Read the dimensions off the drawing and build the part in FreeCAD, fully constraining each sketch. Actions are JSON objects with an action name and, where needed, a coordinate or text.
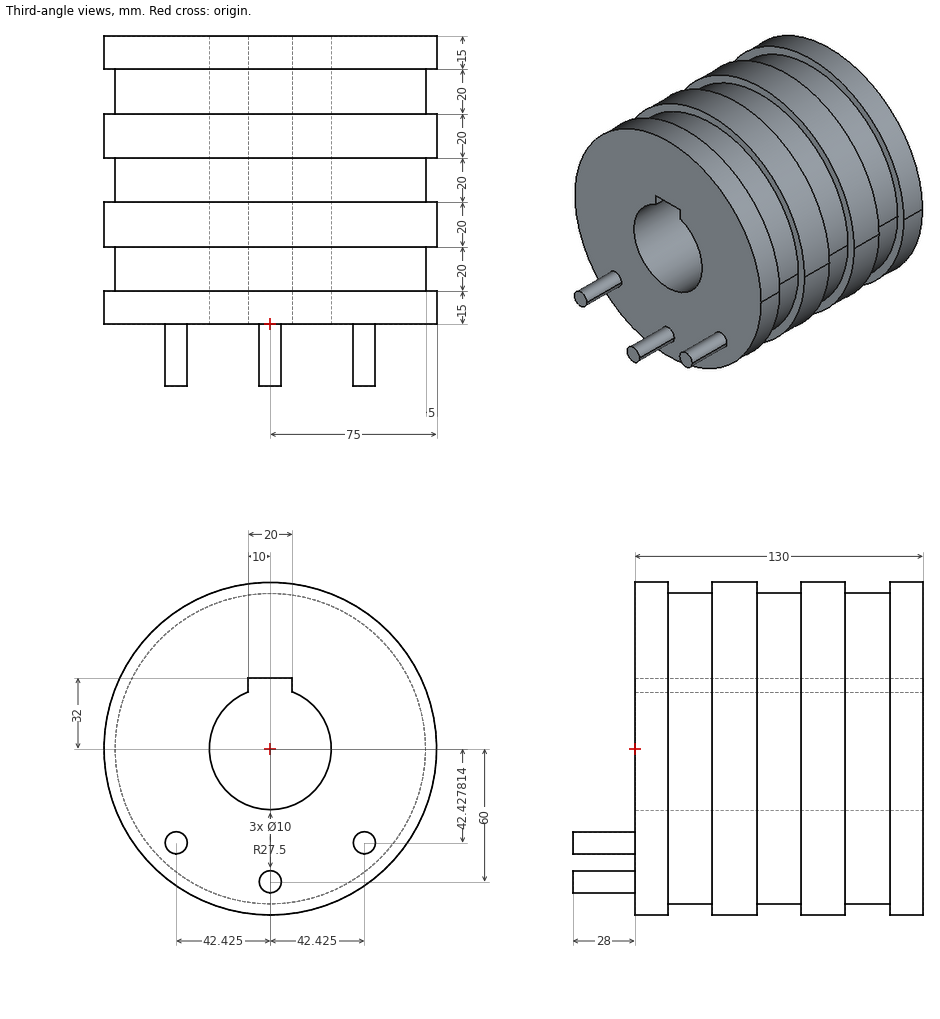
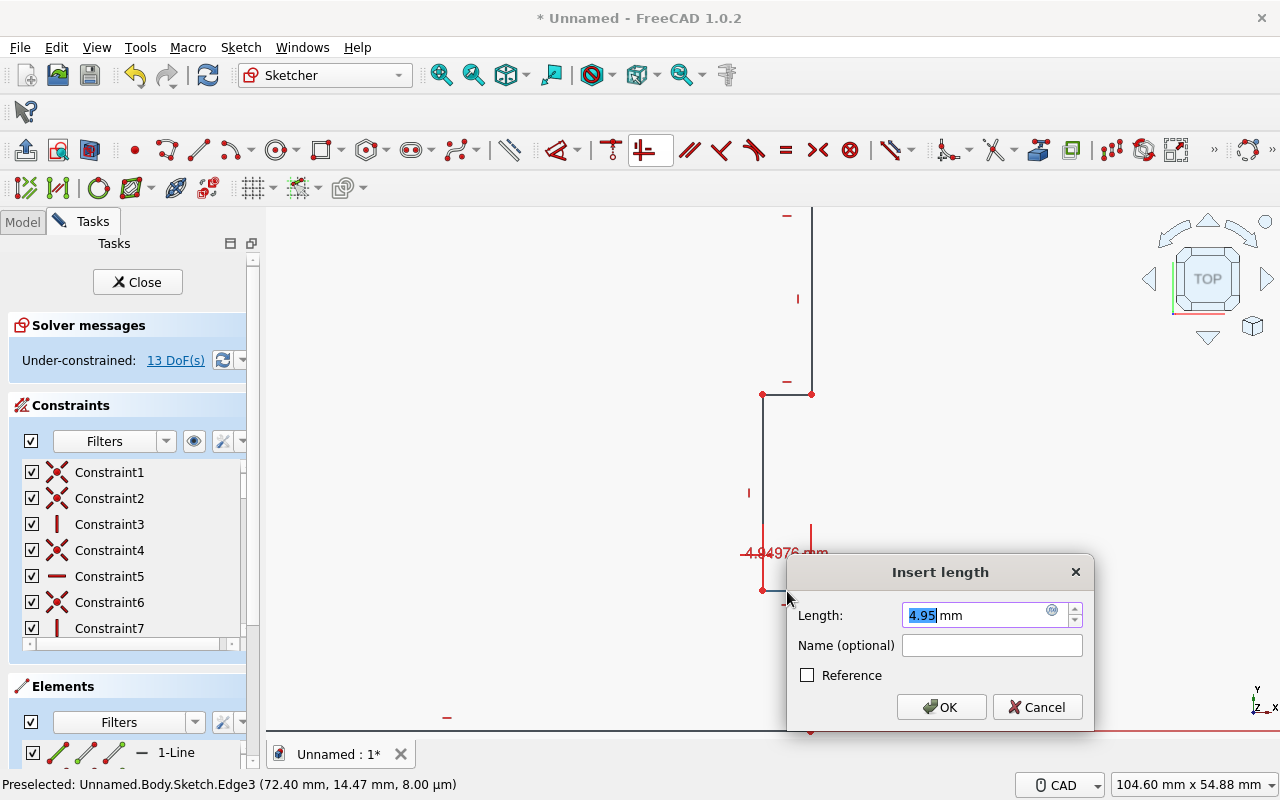
{"action": "type", "text": "5"}
{"action": "key", "text": "Return"}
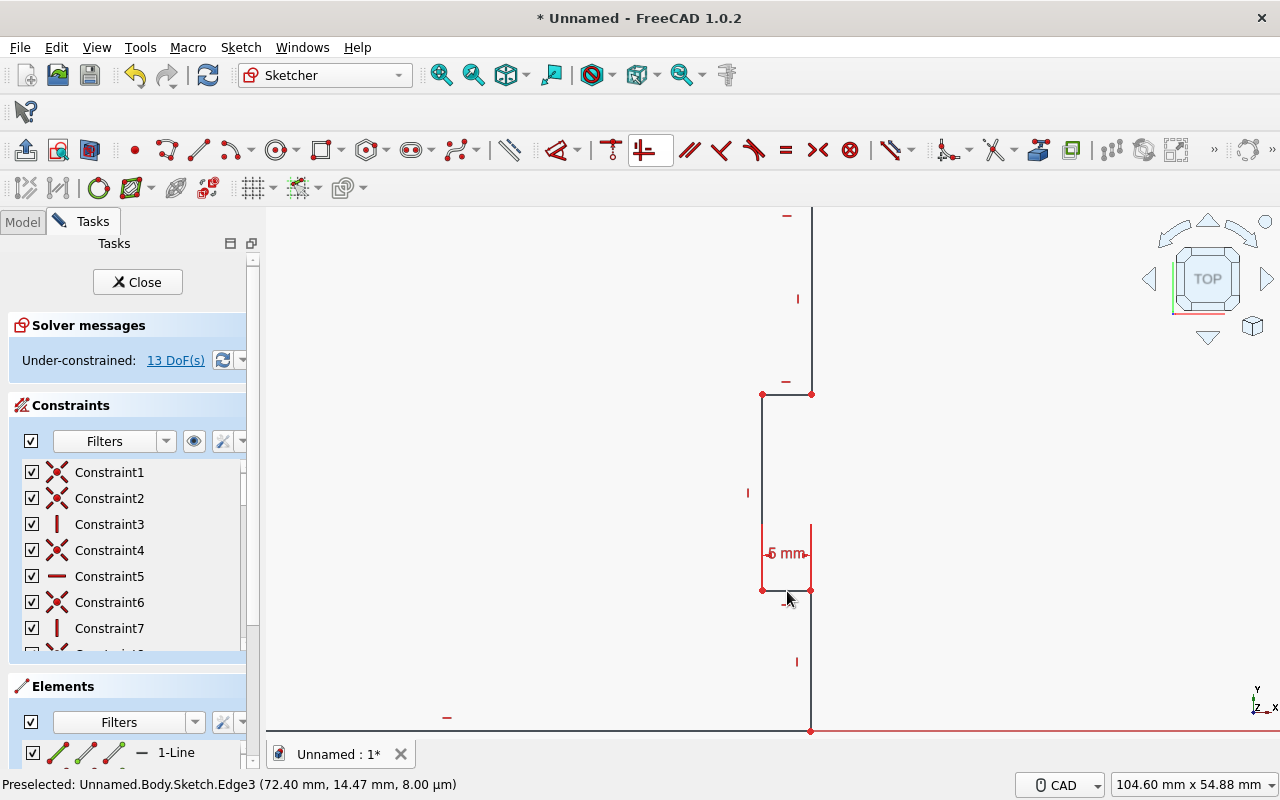
{"action": "left_click", "coordinate": [777, 395]}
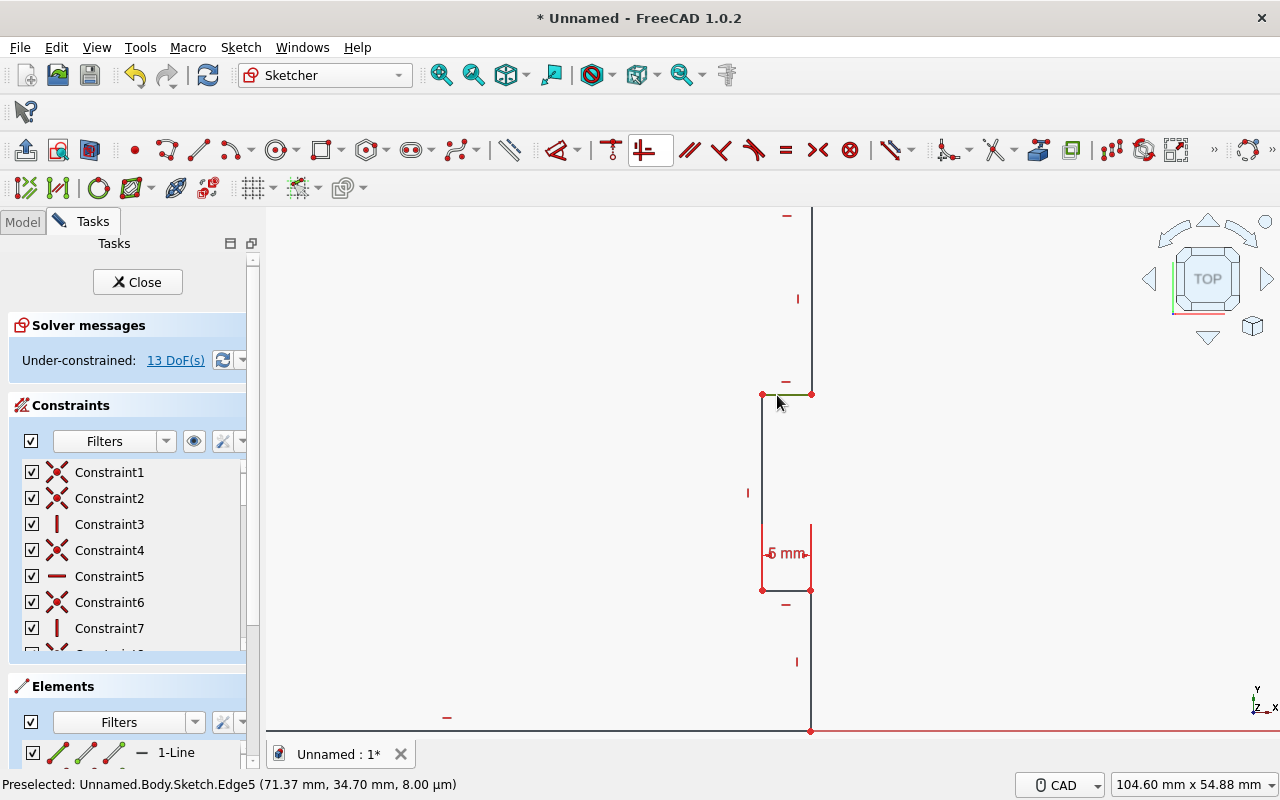
{"action": "left_click", "coordinate": [580, 150]}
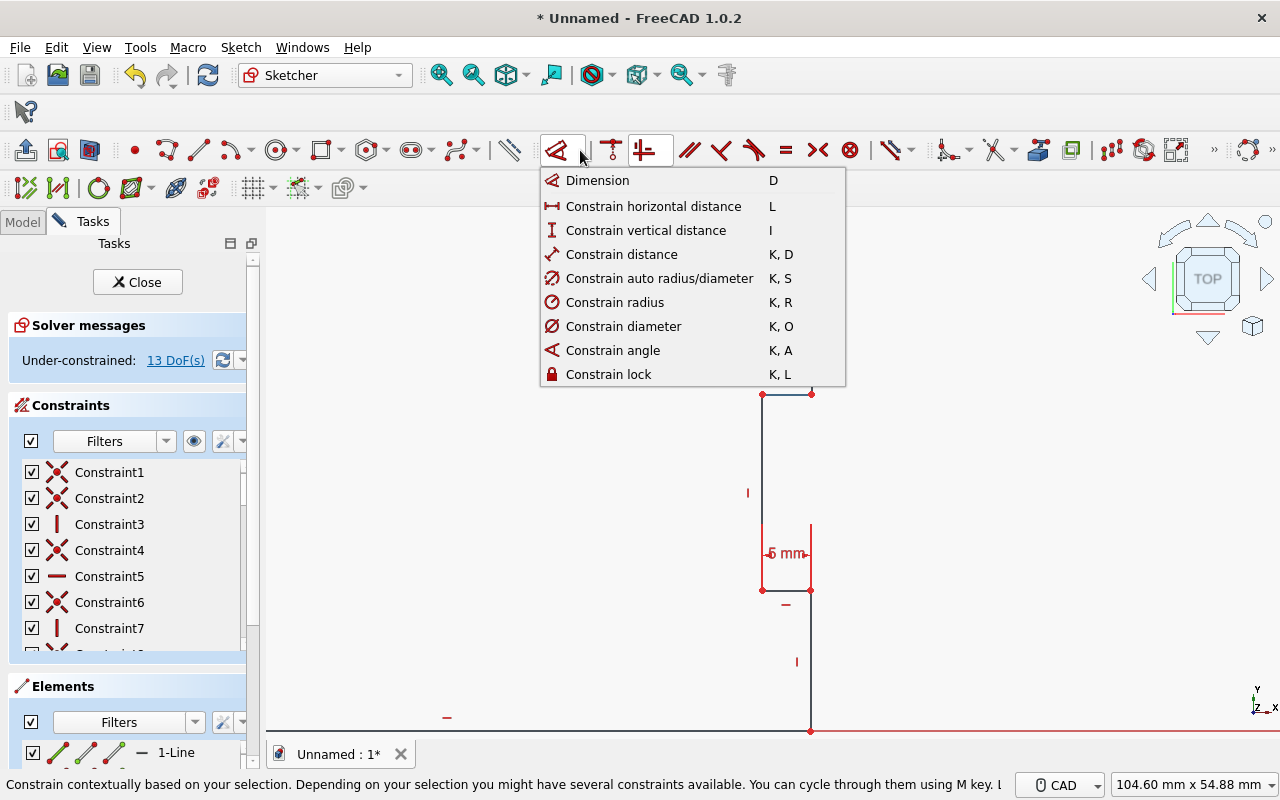
{"action": "left_click", "coordinate": [693, 206]}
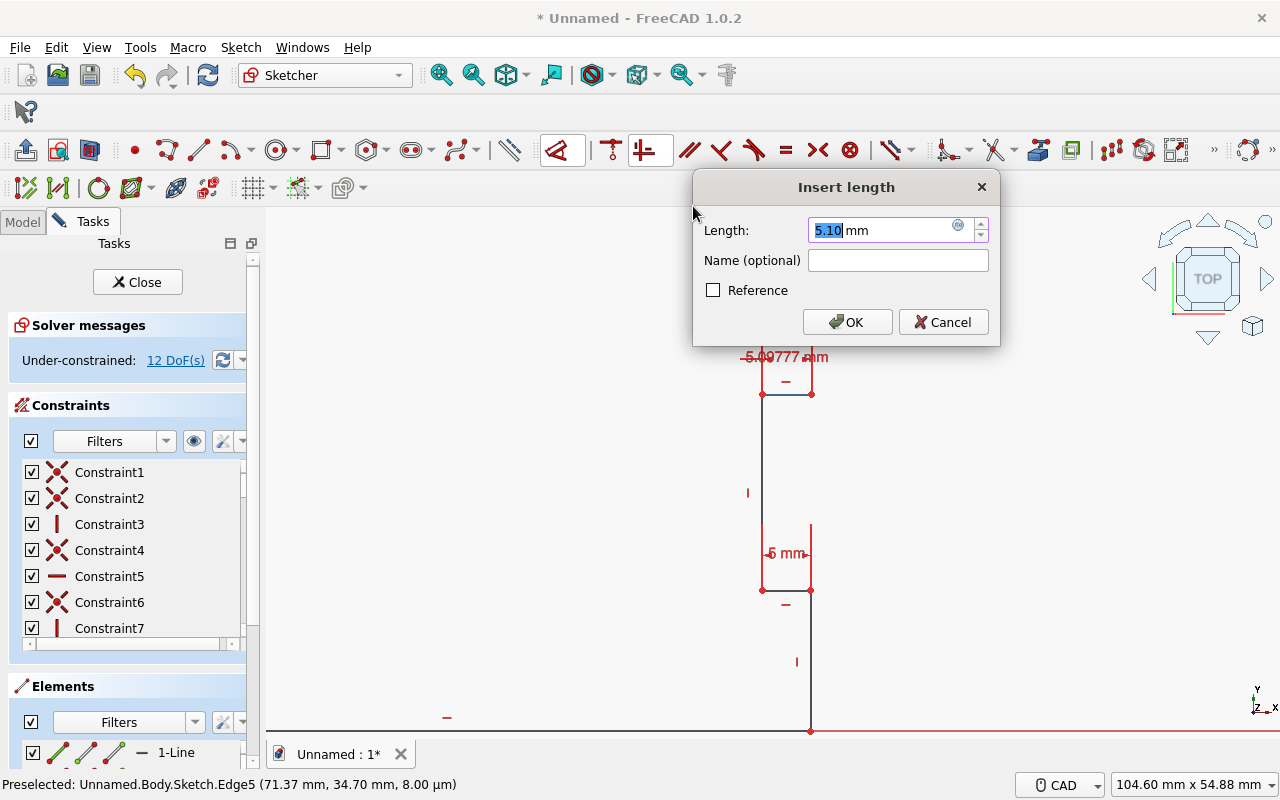
{"action": "type", "text": "5"}
{"action": "key", "text": "Return"}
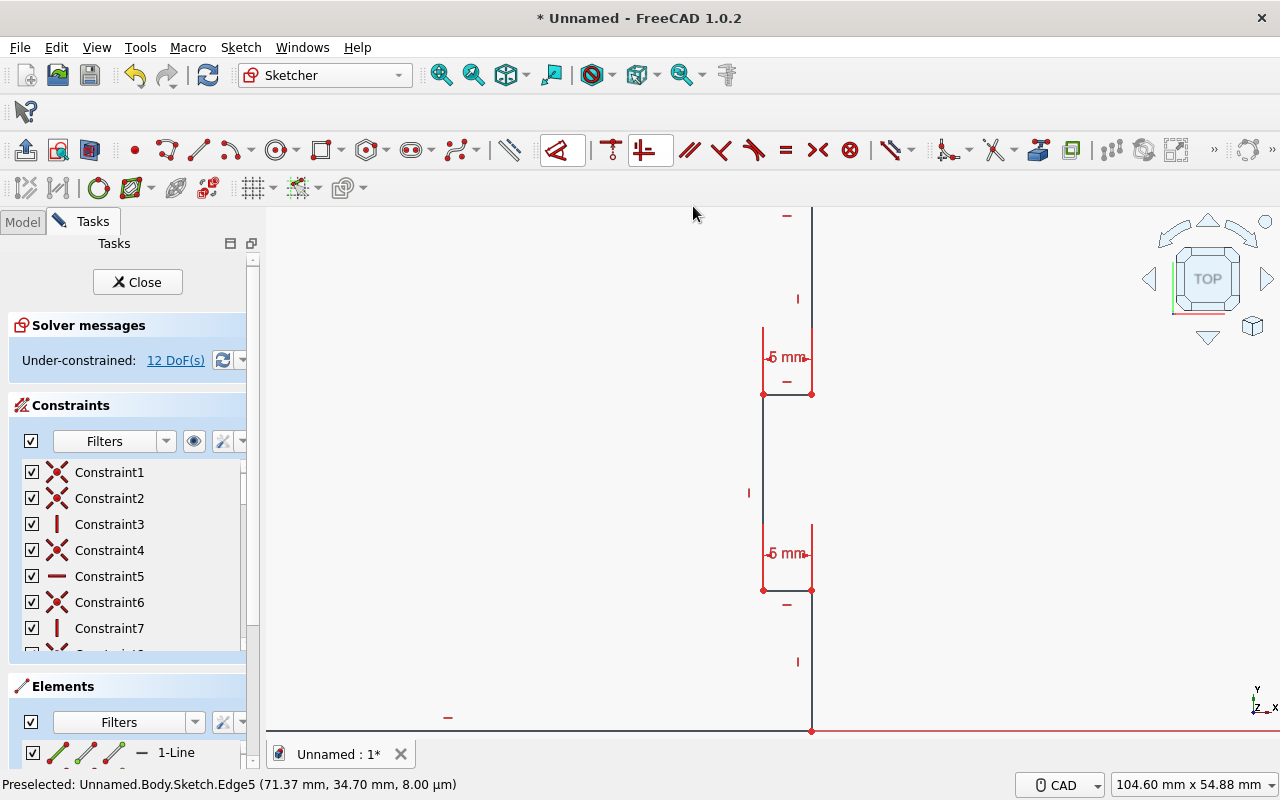
{"action": "scroll", "coordinate": [788, 595], "scroll_direction": "down", "scroll_amount": 7}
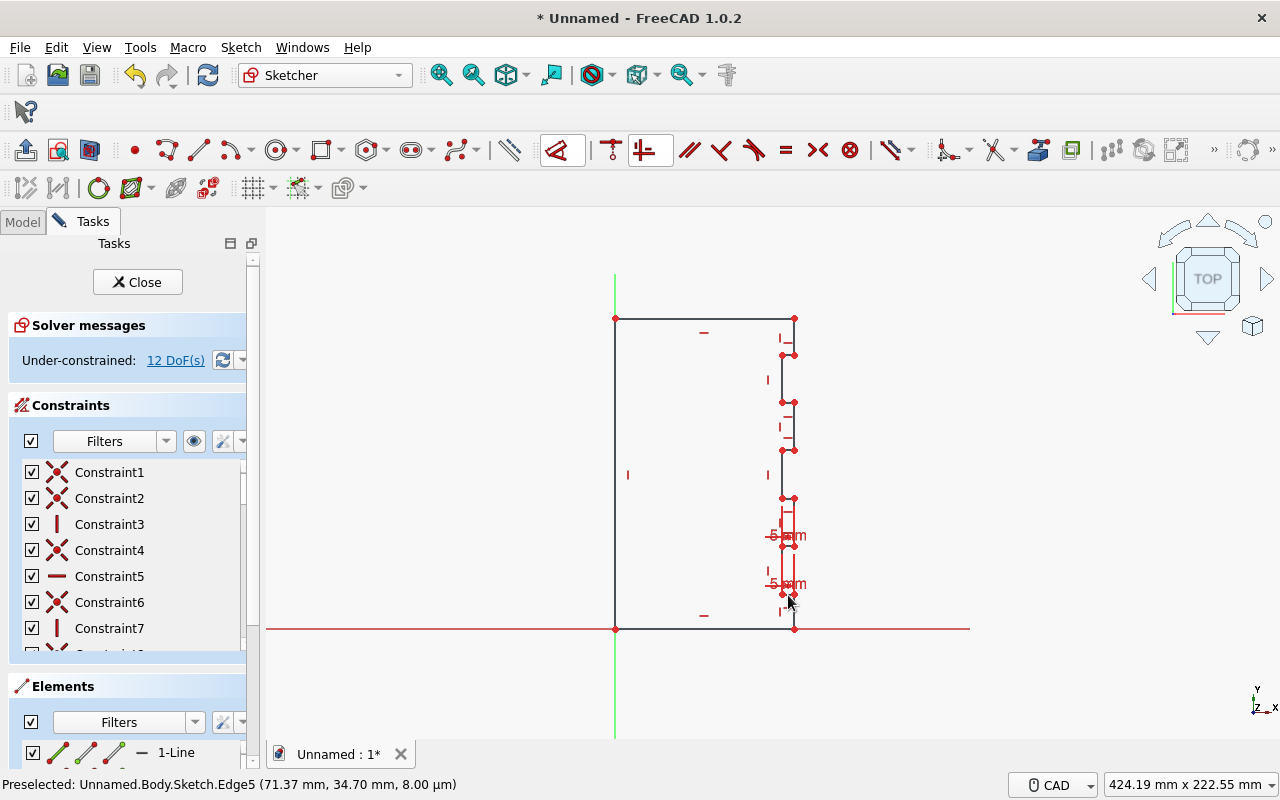
{"action": "scroll", "coordinate": [791, 499], "scroll_direction": "up", "scroll_amount": 7}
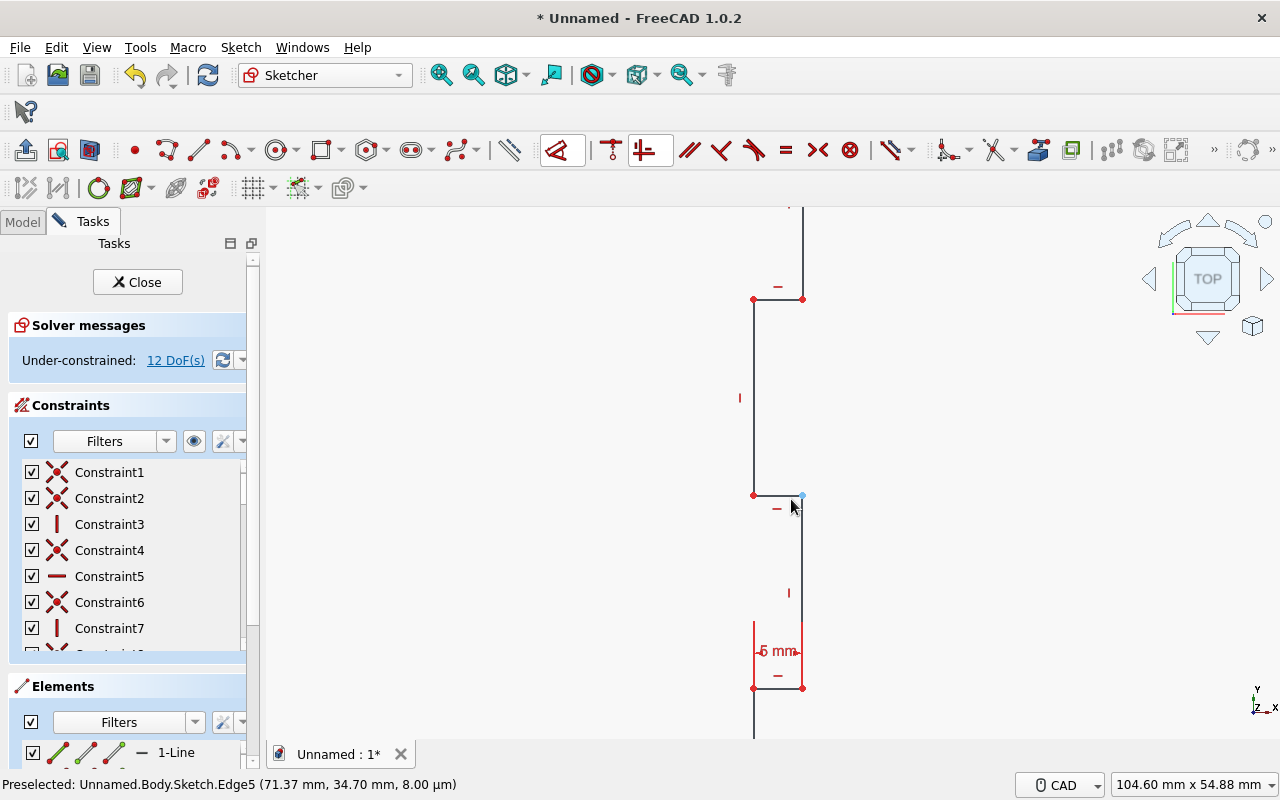
{"action": "left_click", "coordinate": [788, 496]}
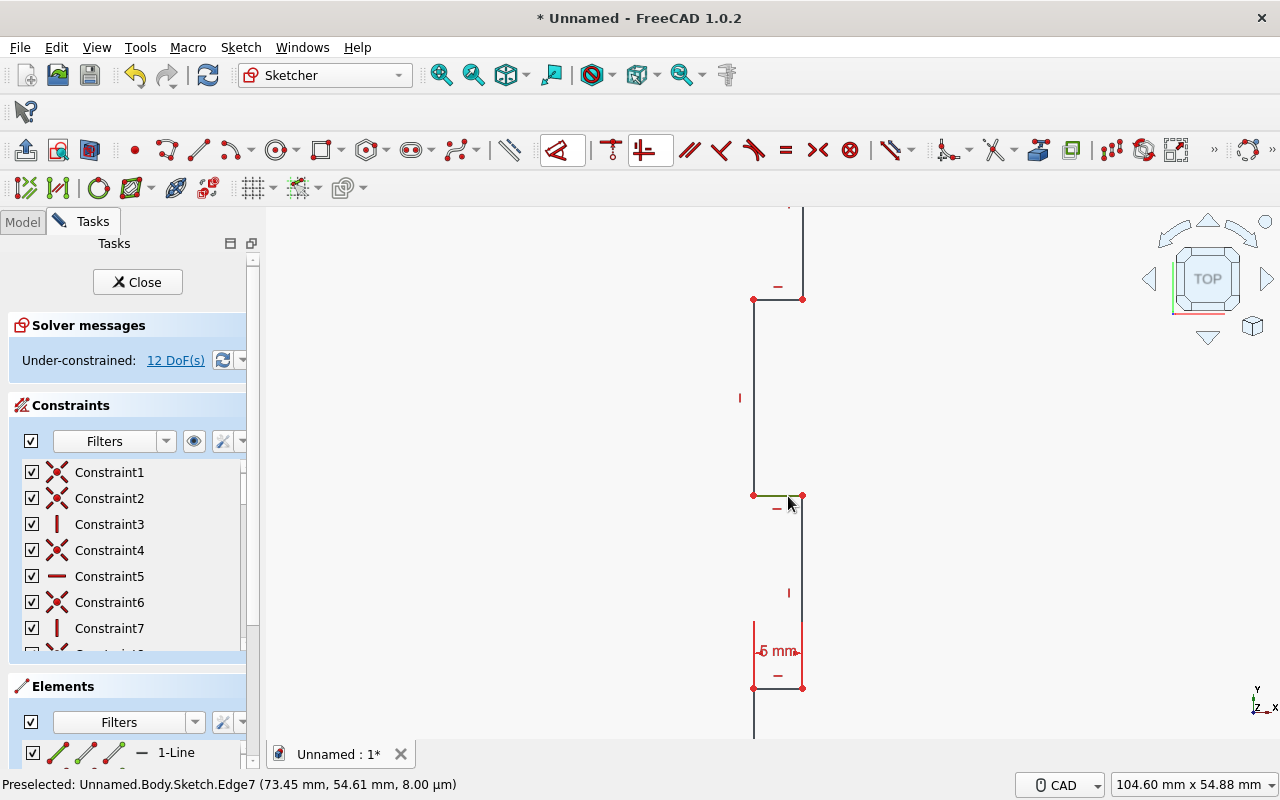
{"action": "key", "text": "l"}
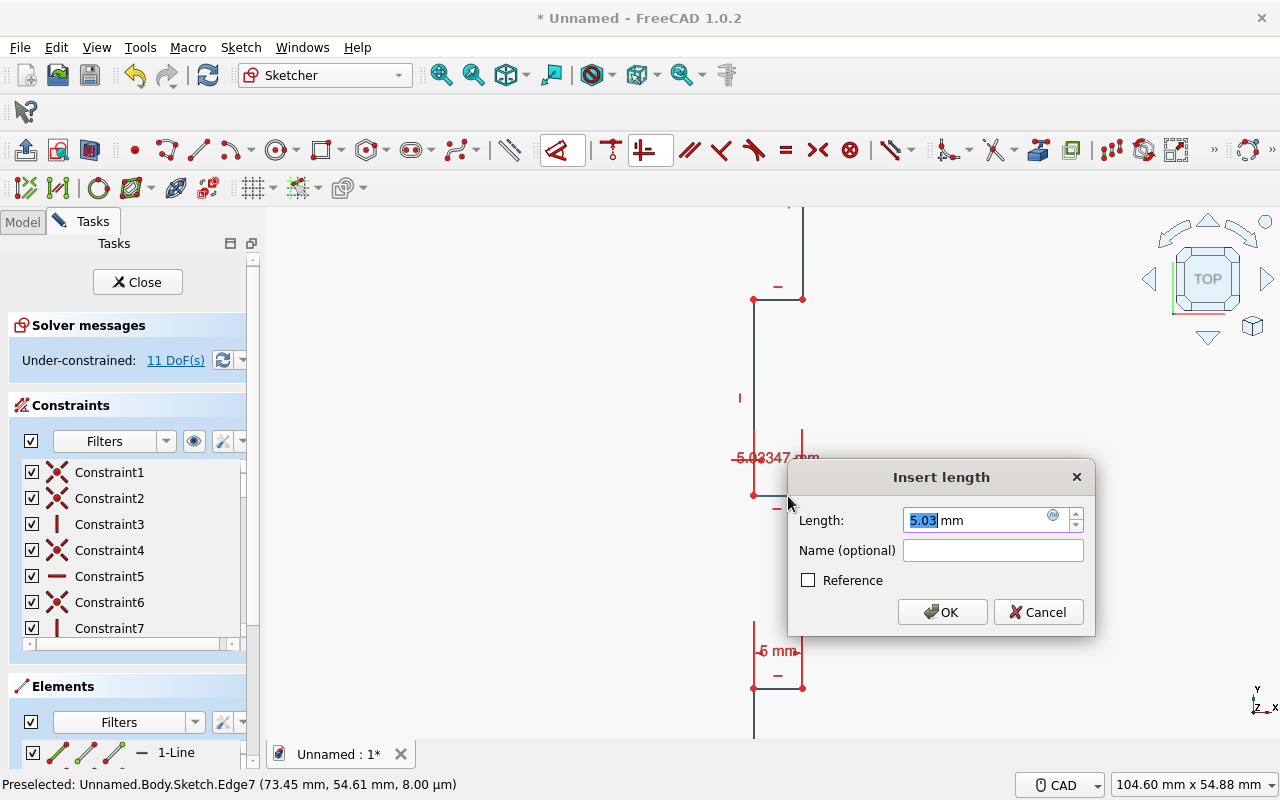
{"action": "type", "text": "5"}
{"action": "key", "text": "Return"}